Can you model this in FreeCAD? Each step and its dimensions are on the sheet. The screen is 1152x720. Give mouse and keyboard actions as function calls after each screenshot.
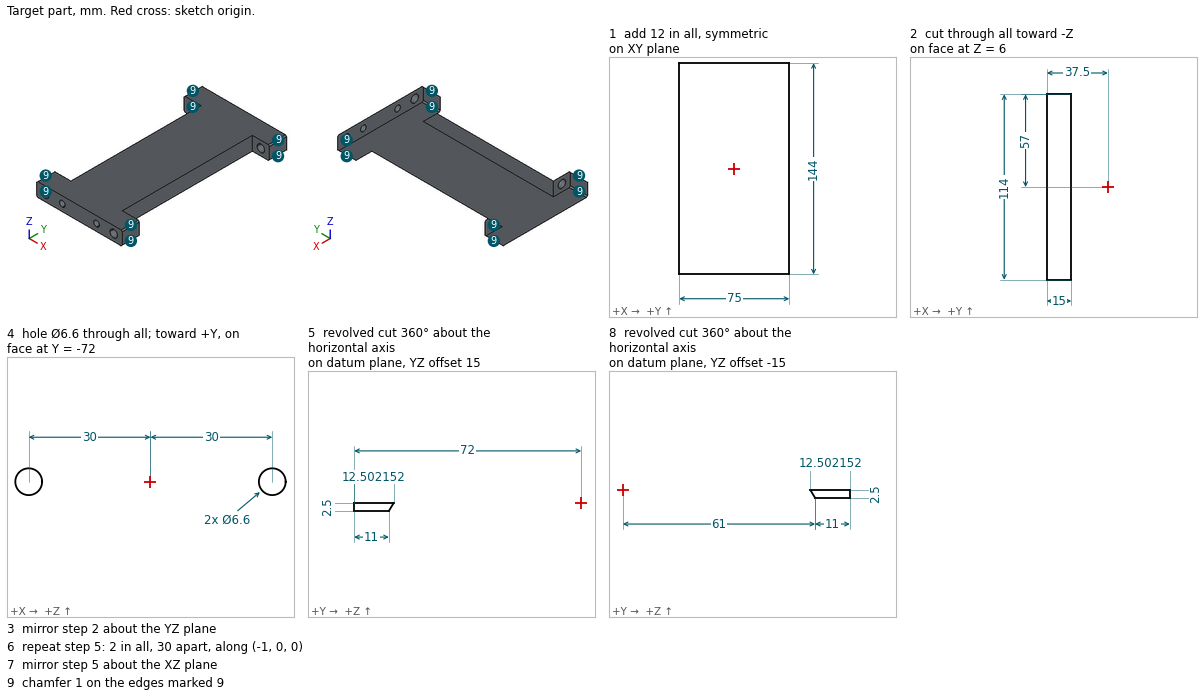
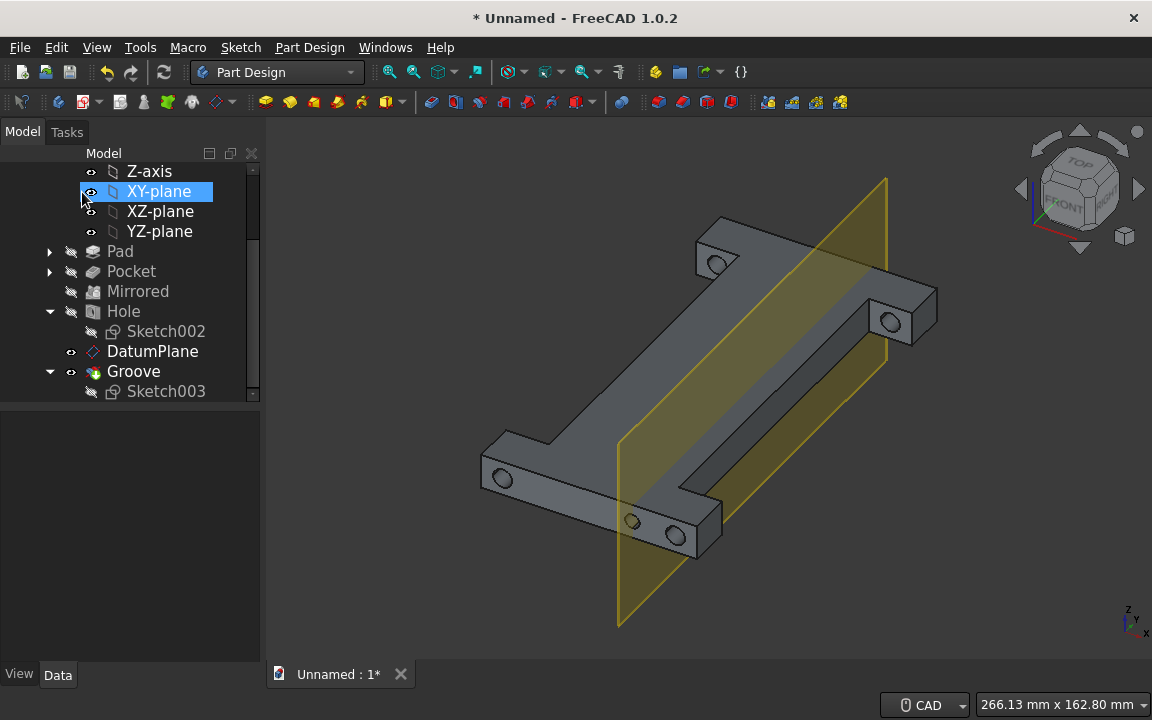
click(116, 352)
key(space)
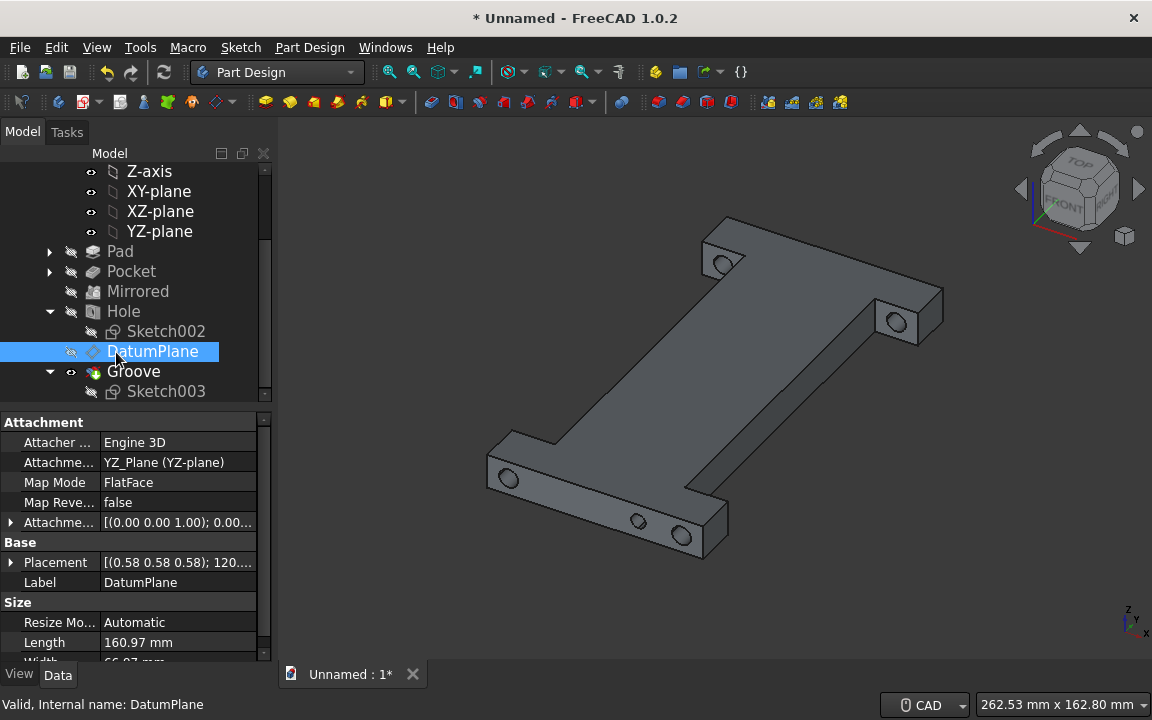
click(116, 372)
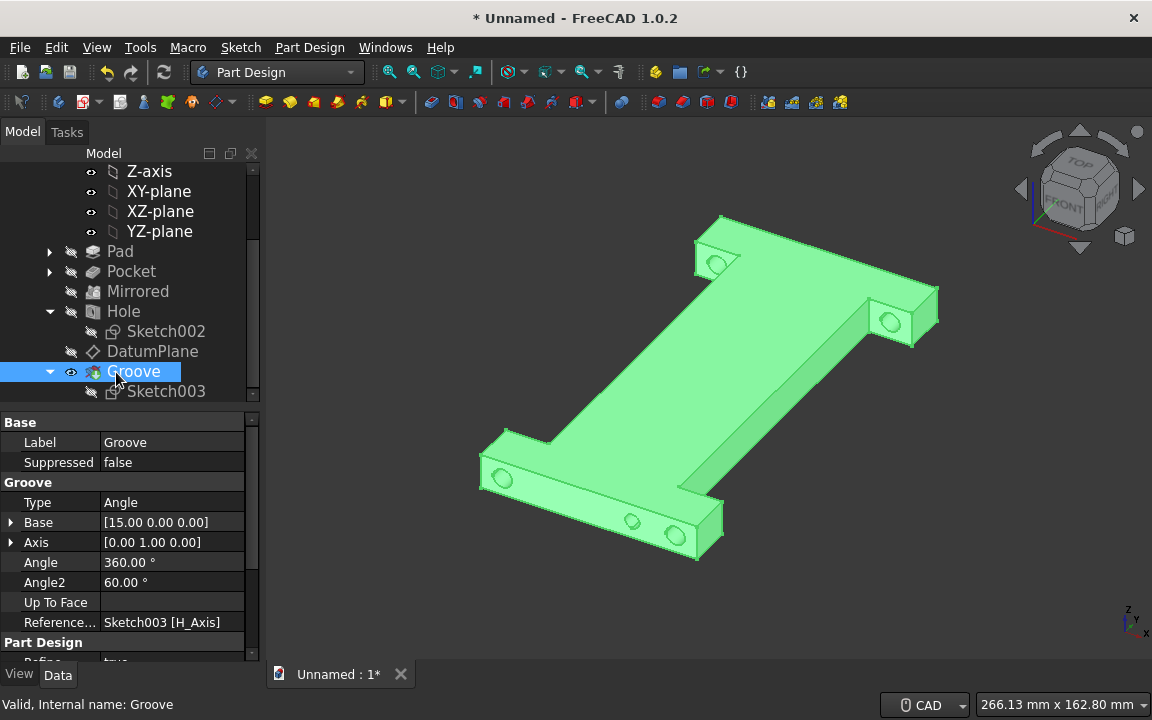
click(792, 102)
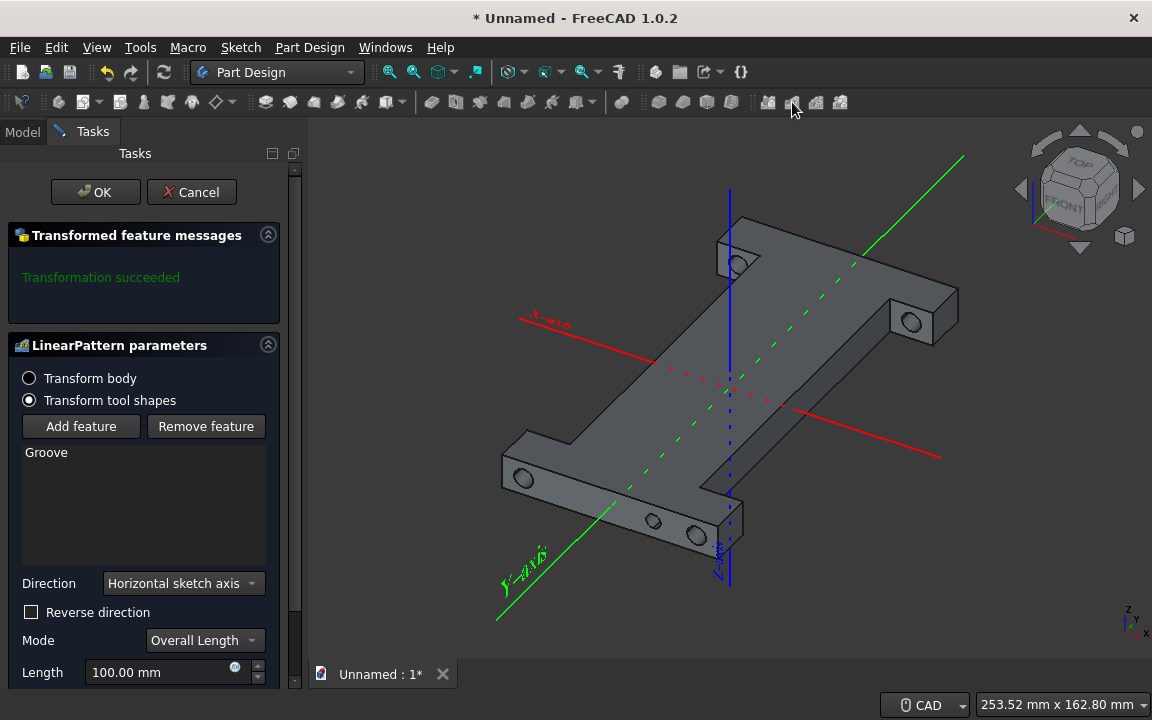
click(184, 584)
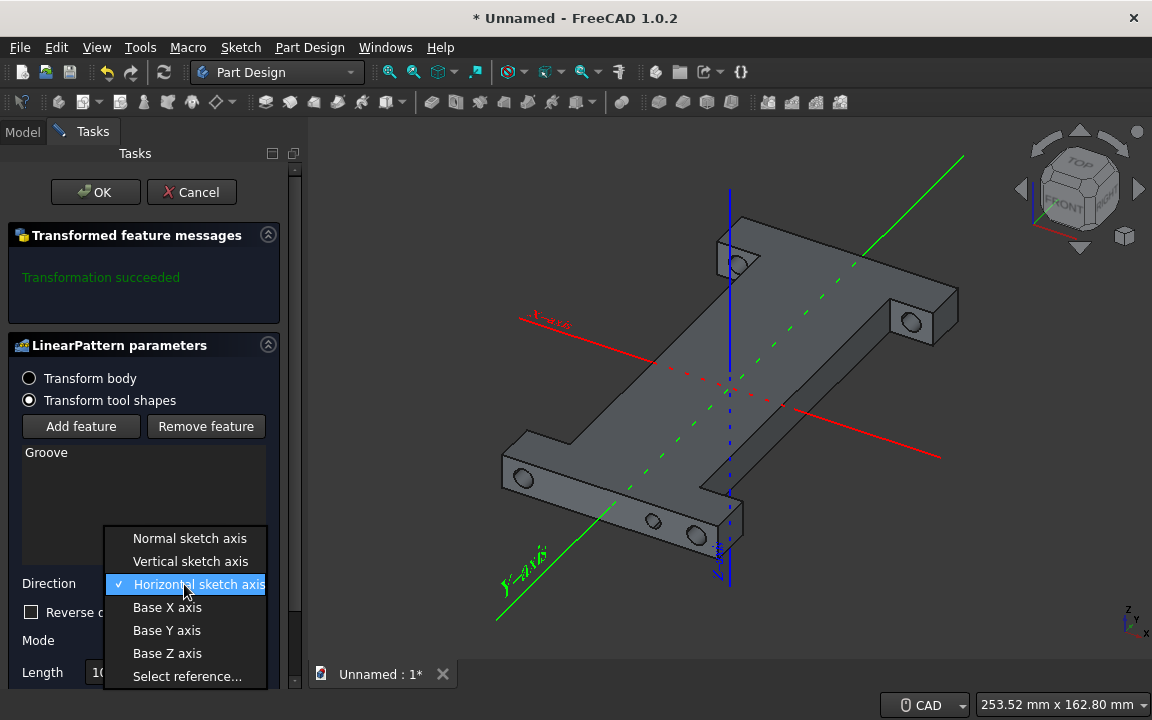
click(184, 608)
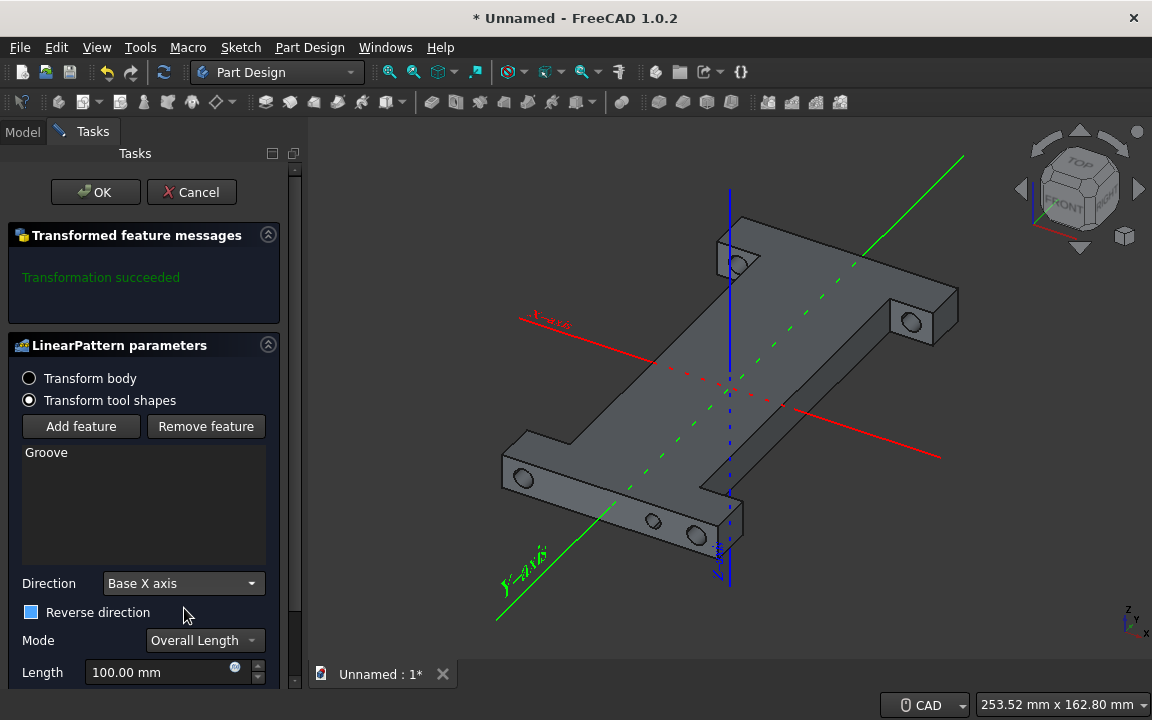
click(206, 640)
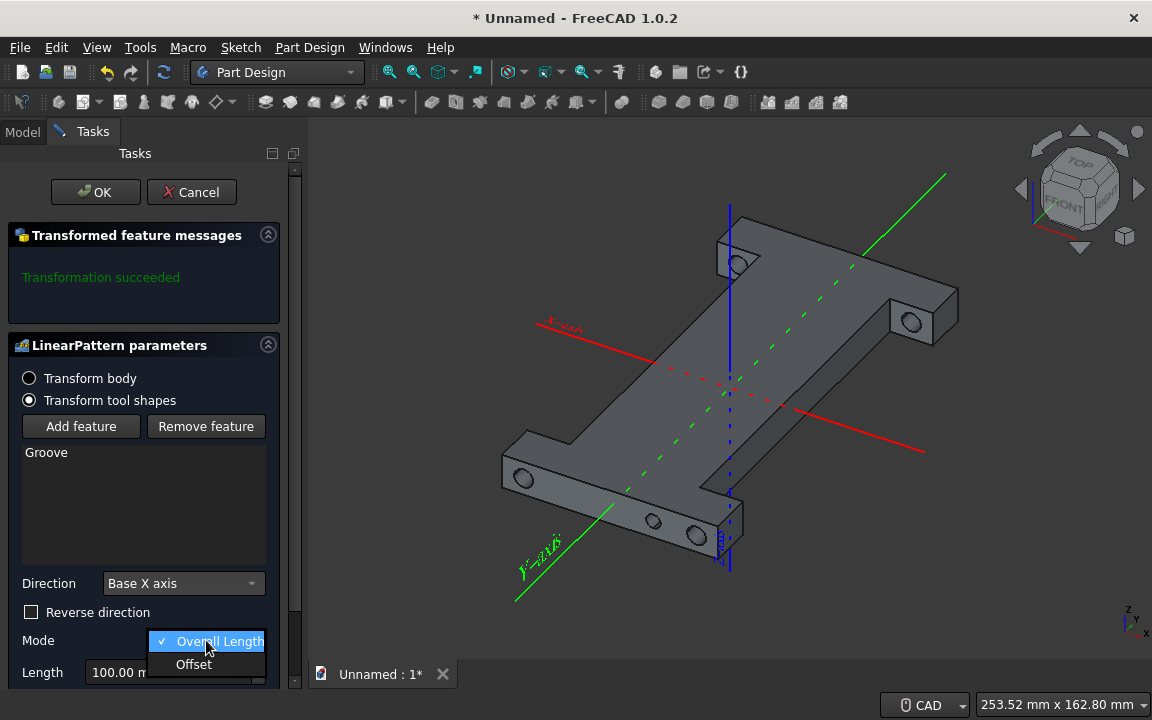
click(206, 664)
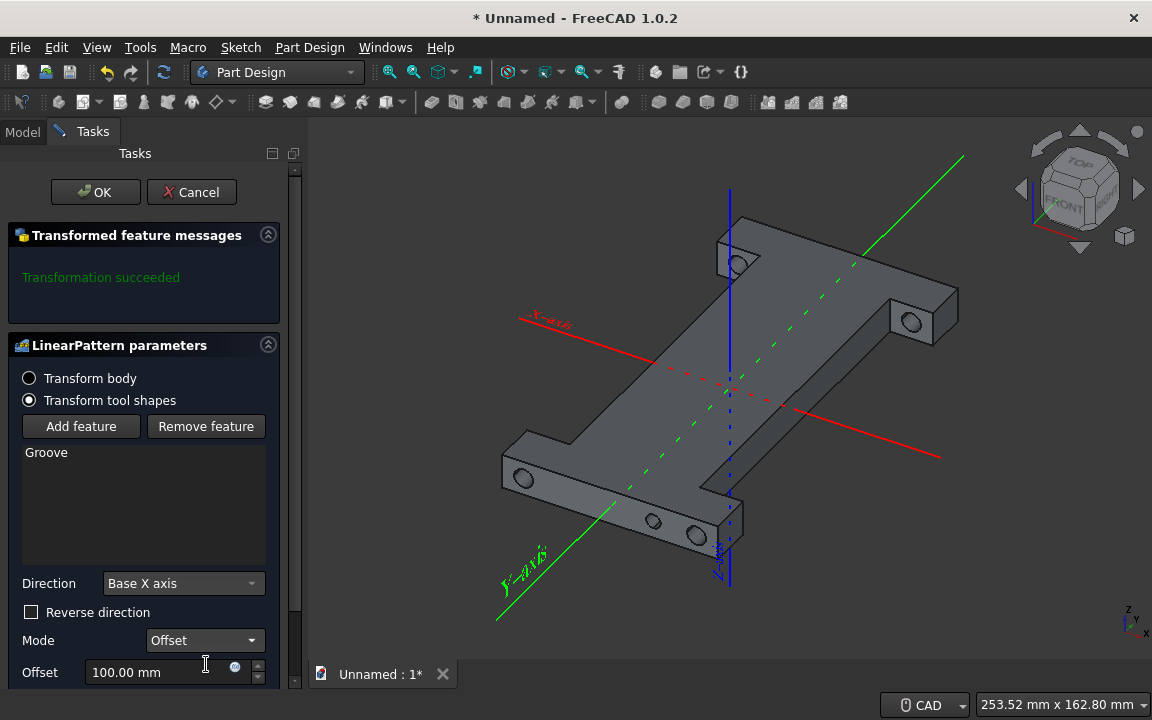
triple_click(168, 672)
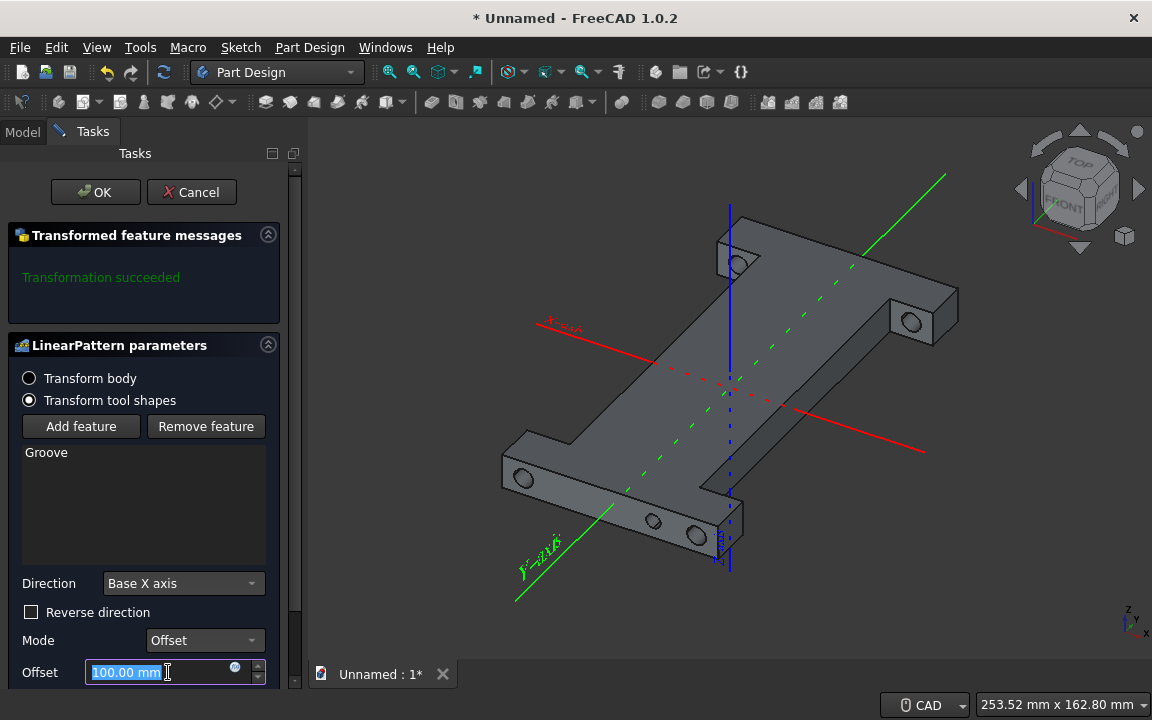
text(30)
key(Tab)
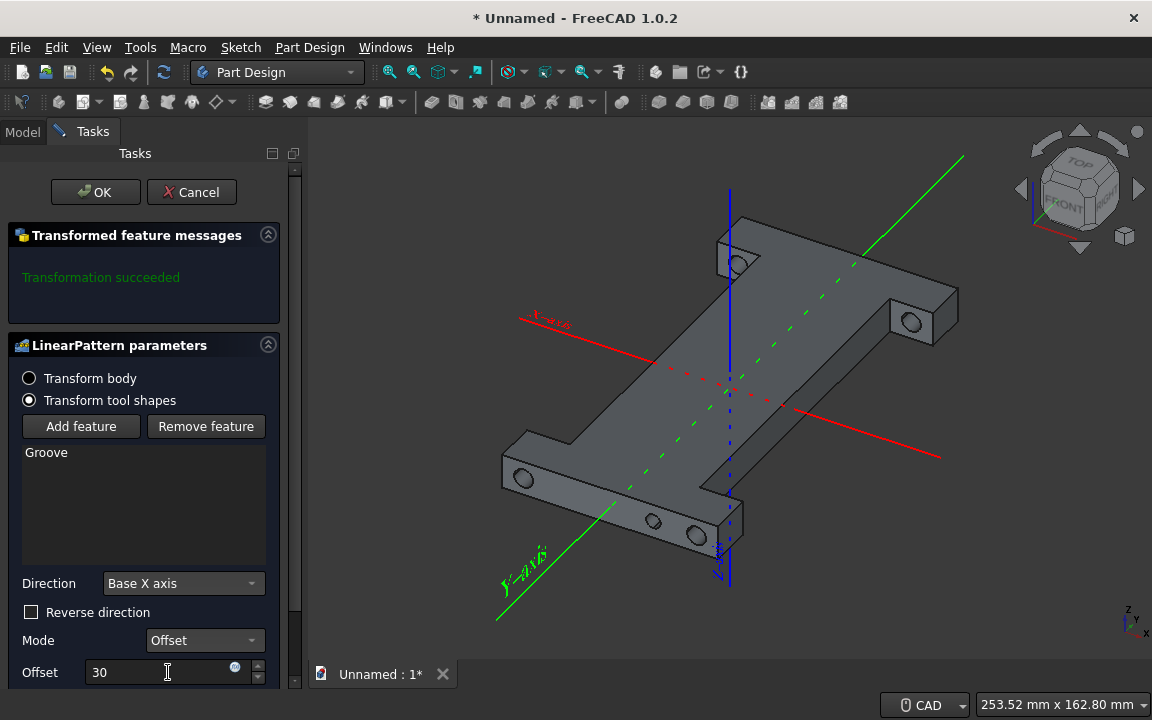
scroll(295, 426, down, 2)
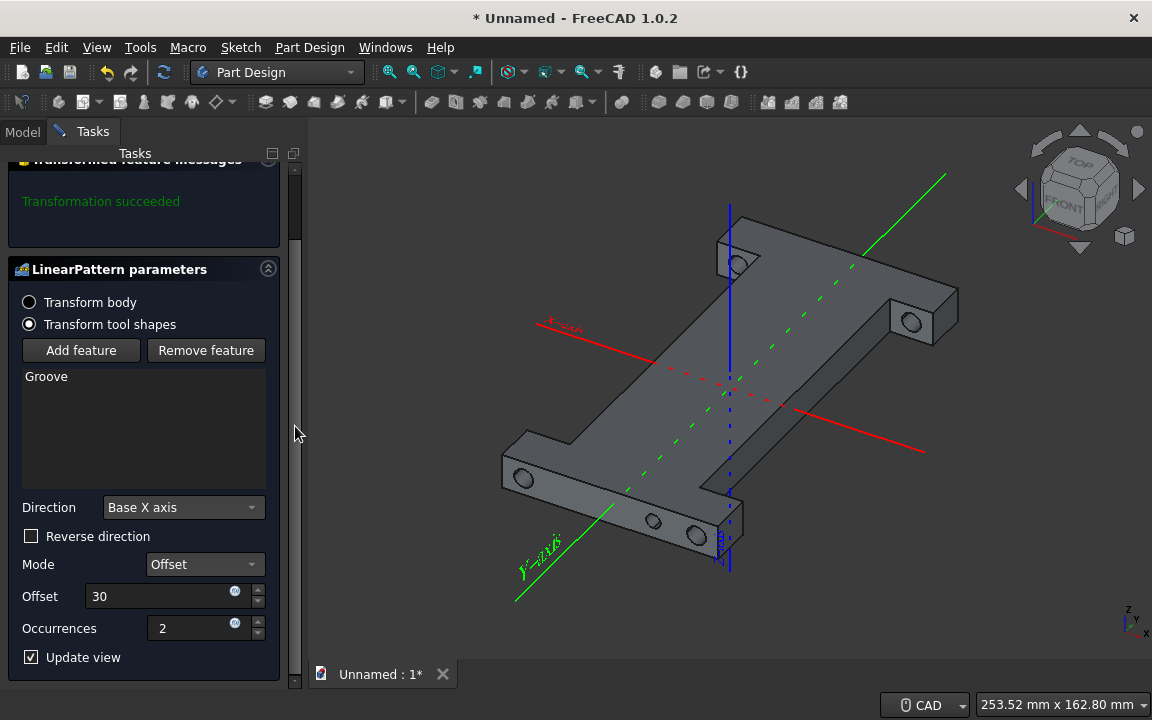
triple_click(198, 628)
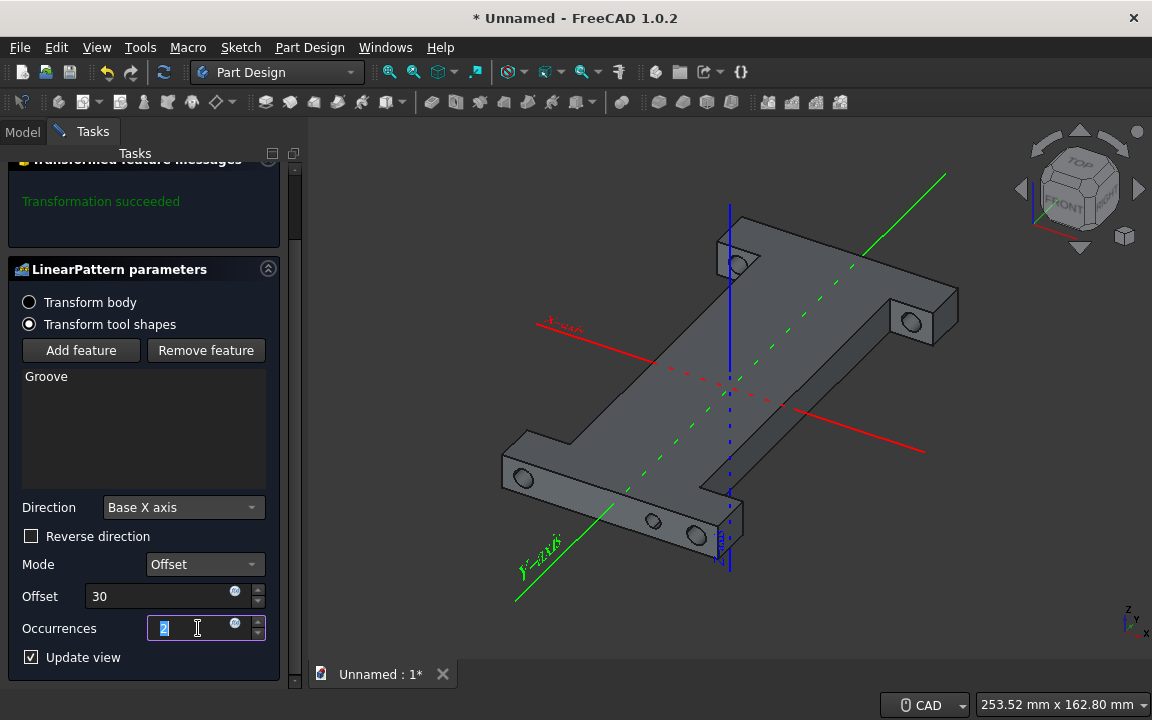
text(2)
key(Tab)